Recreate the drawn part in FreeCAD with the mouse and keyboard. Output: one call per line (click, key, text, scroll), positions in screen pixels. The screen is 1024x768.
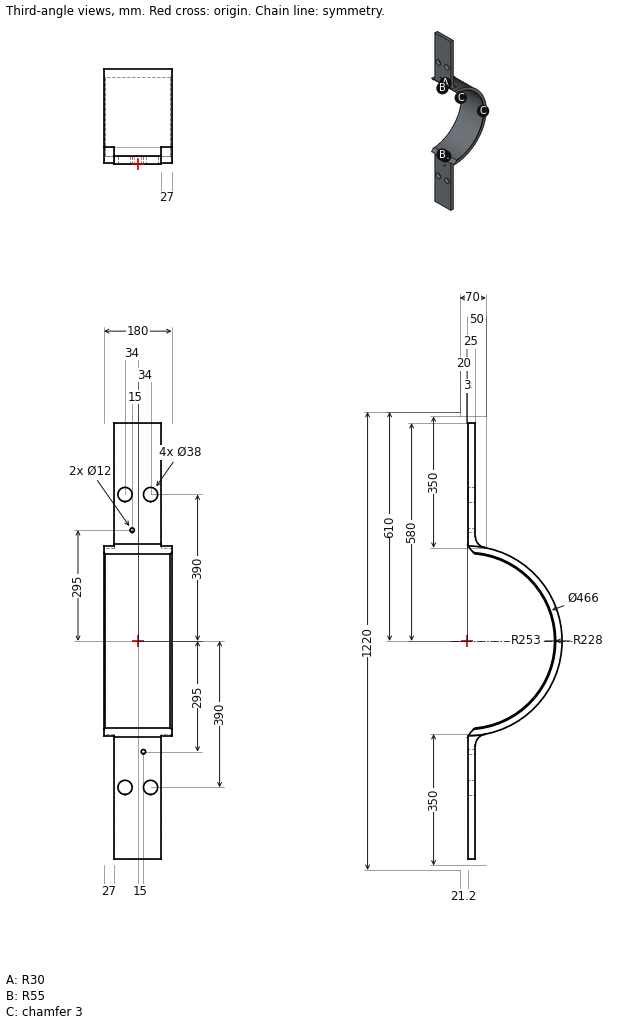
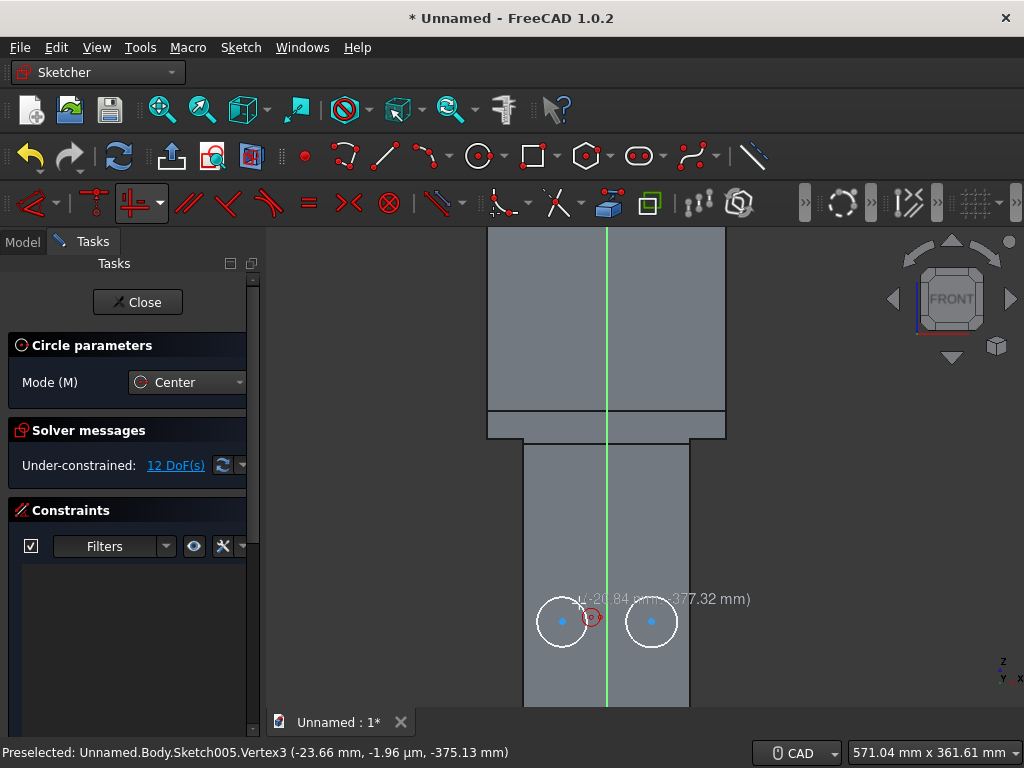
scroll(563, 624, down, 6)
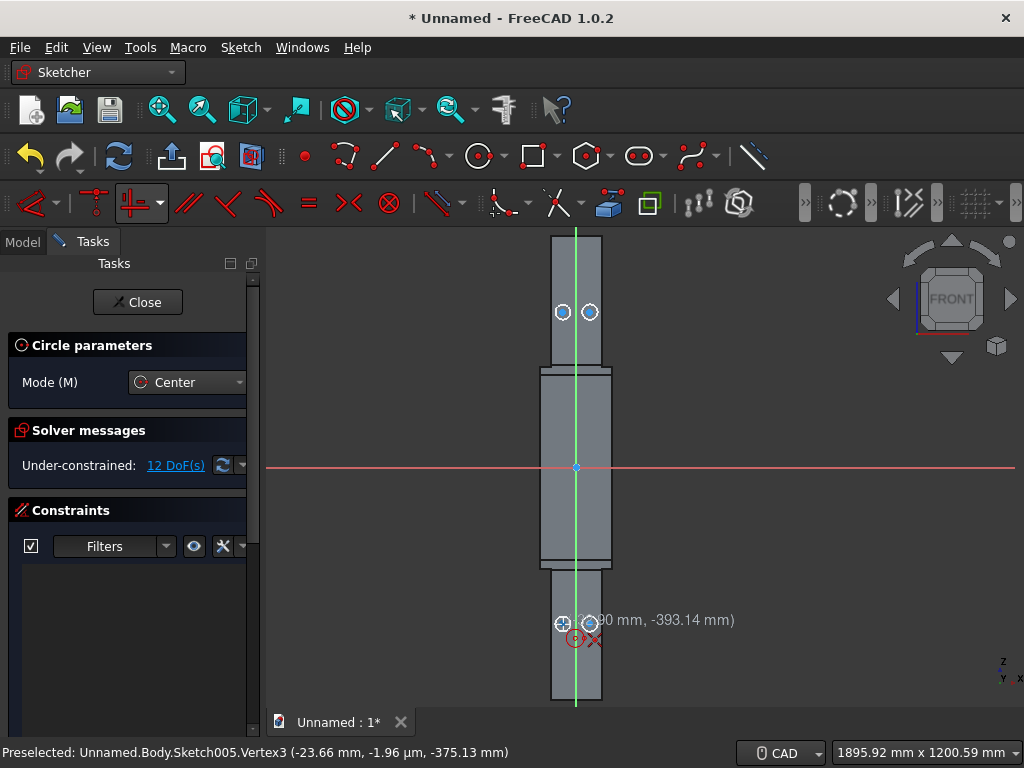
scroll(570, 350, up, 12)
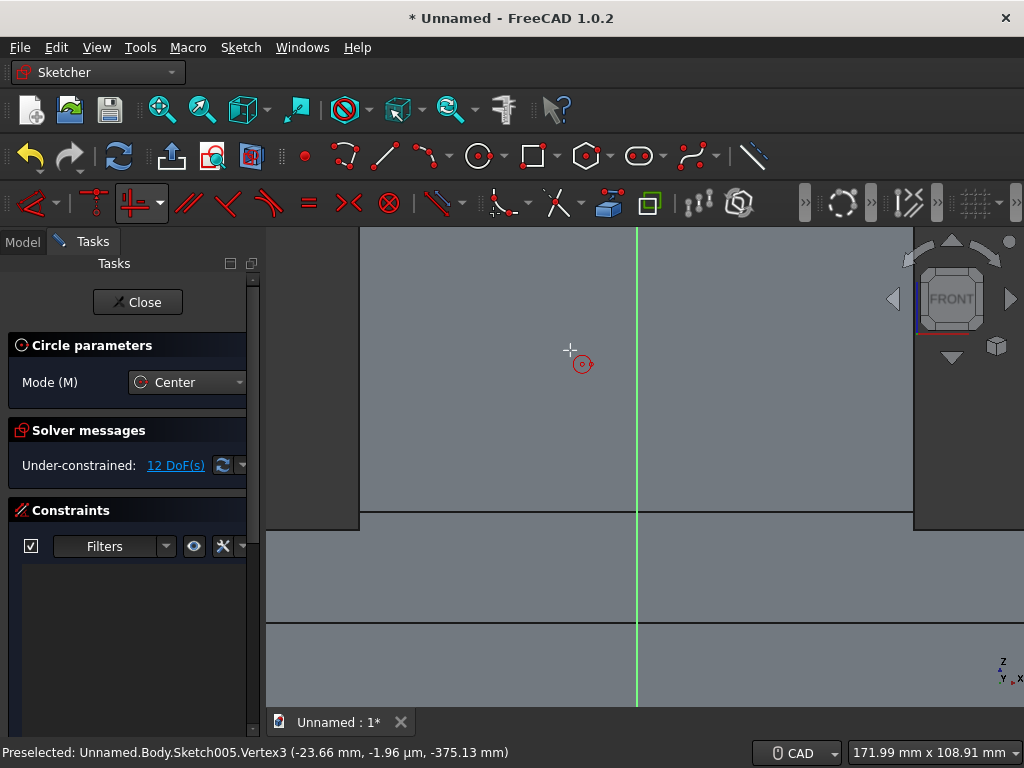
scroll(570, 349, down, 12)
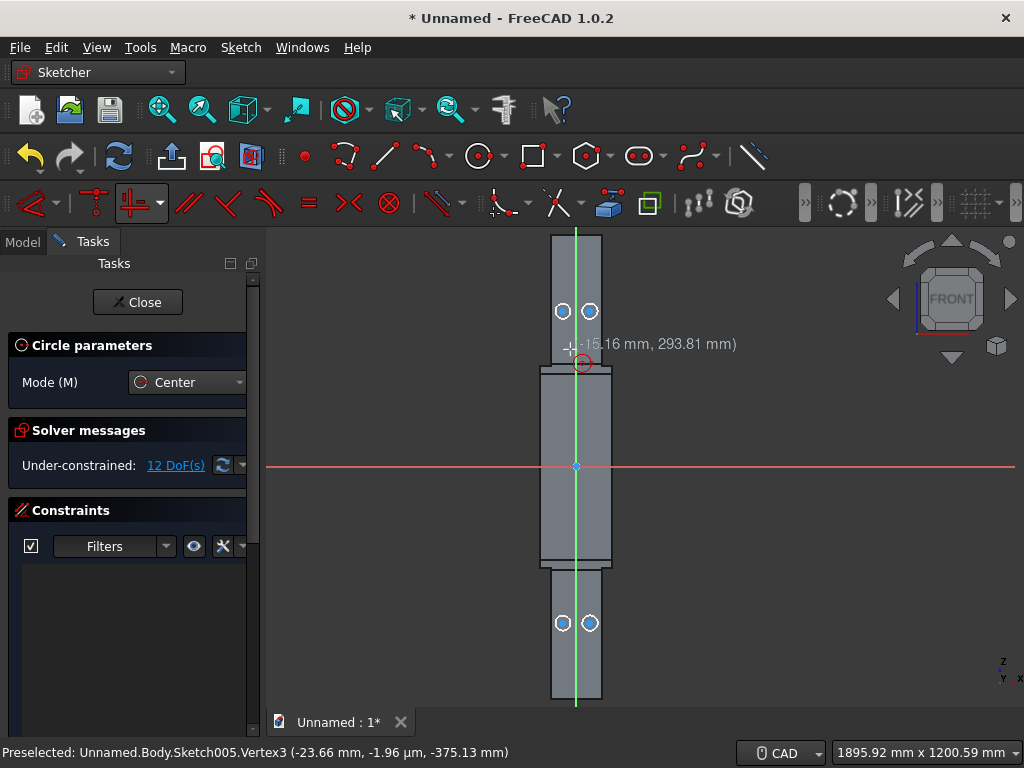
scroll(570, 349, up, 5)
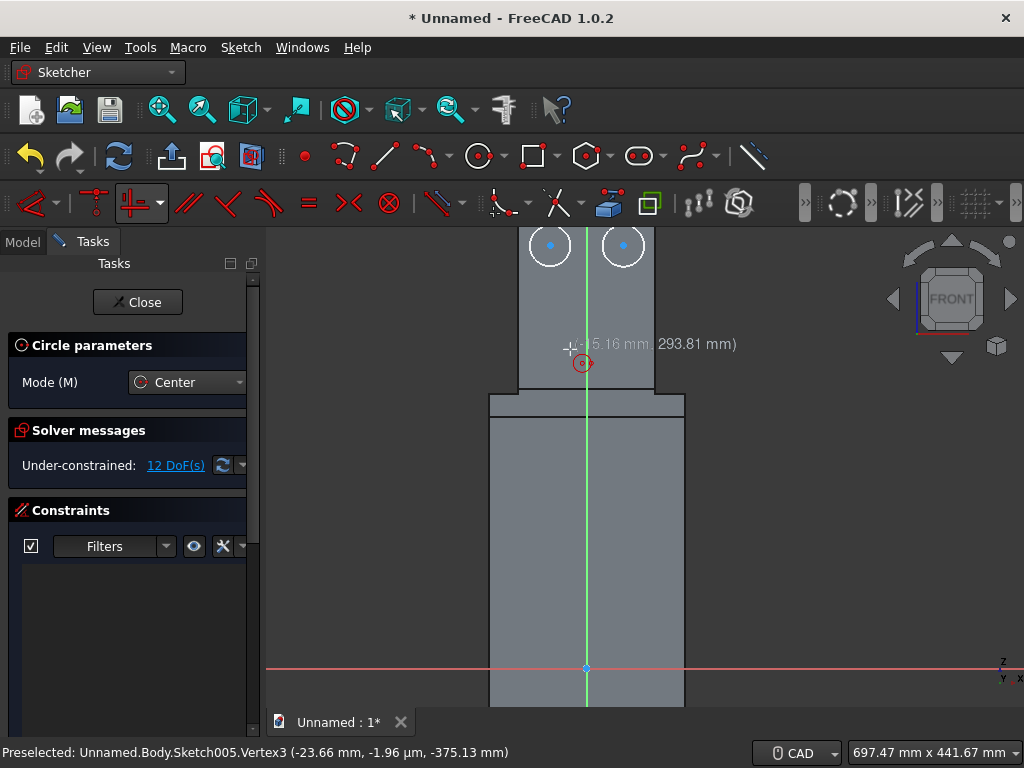
click(570, 348)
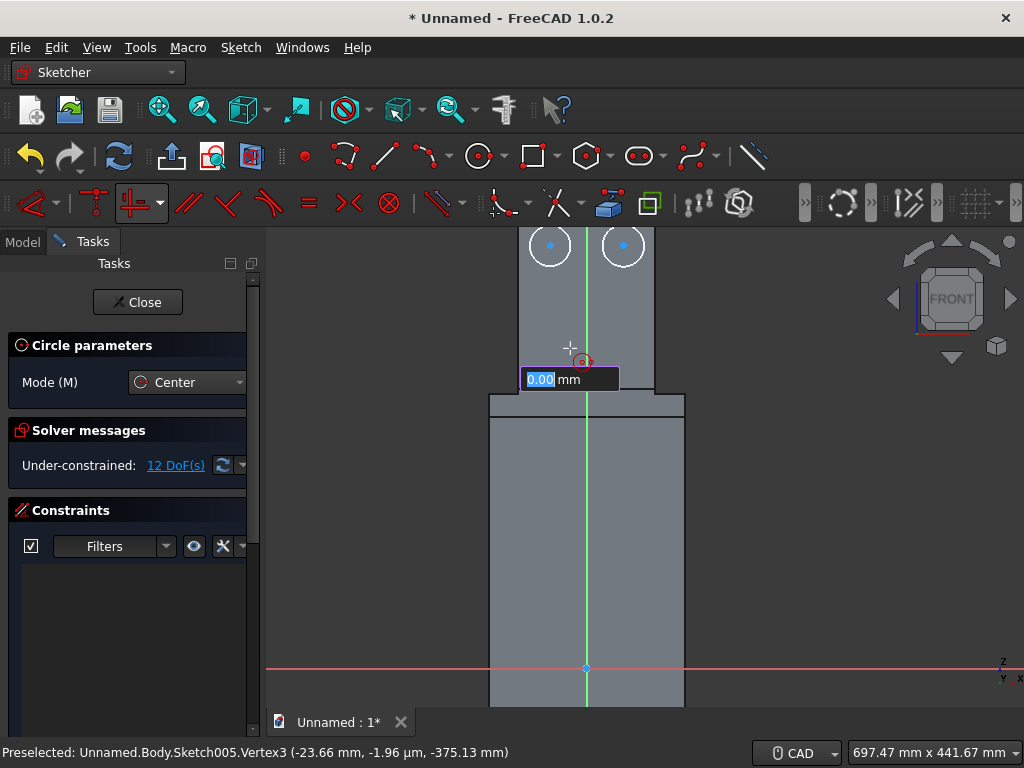
scroll(566, 344, up, 5)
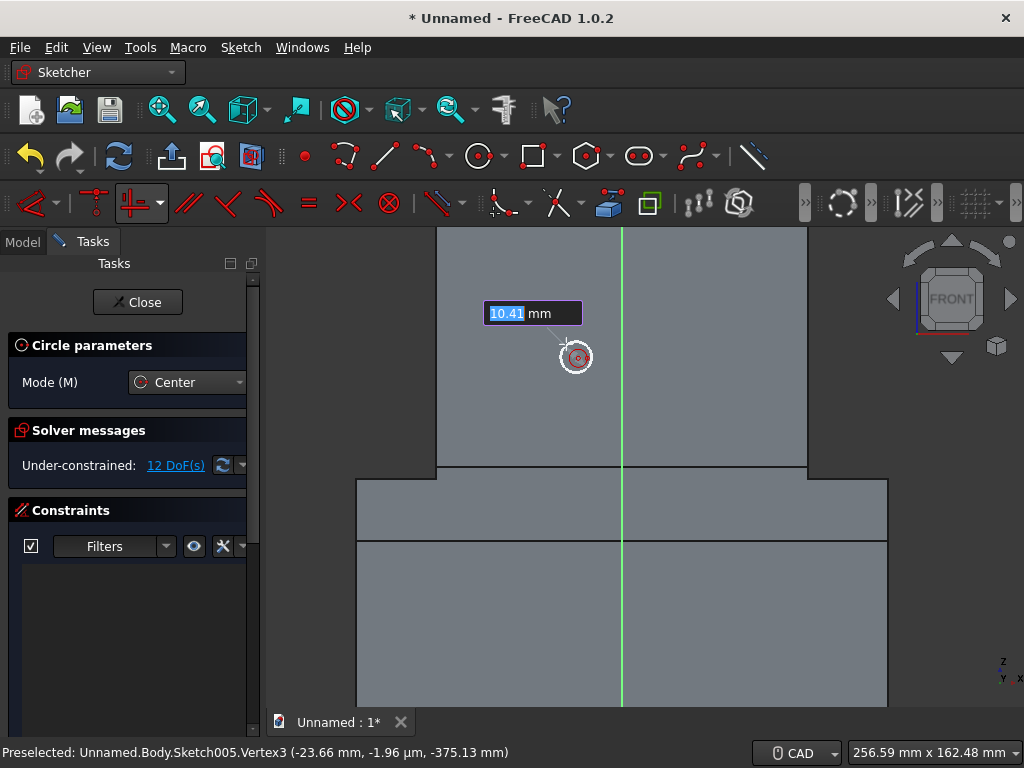
click(565, 342)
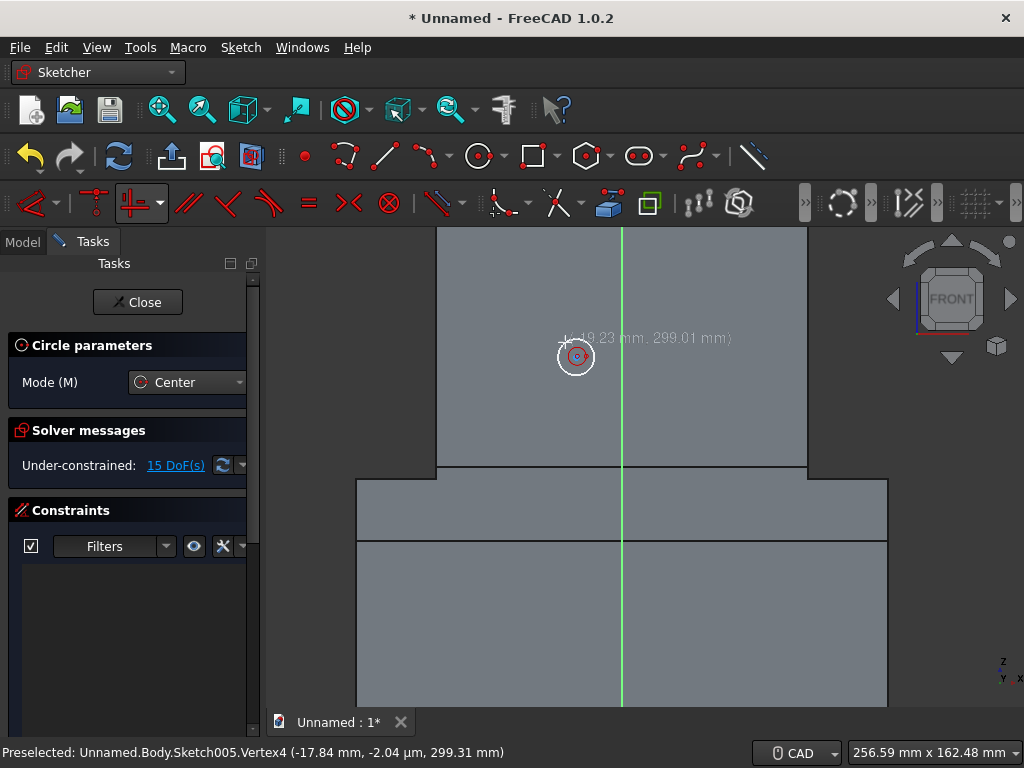
scroll(569, 348, down, 10)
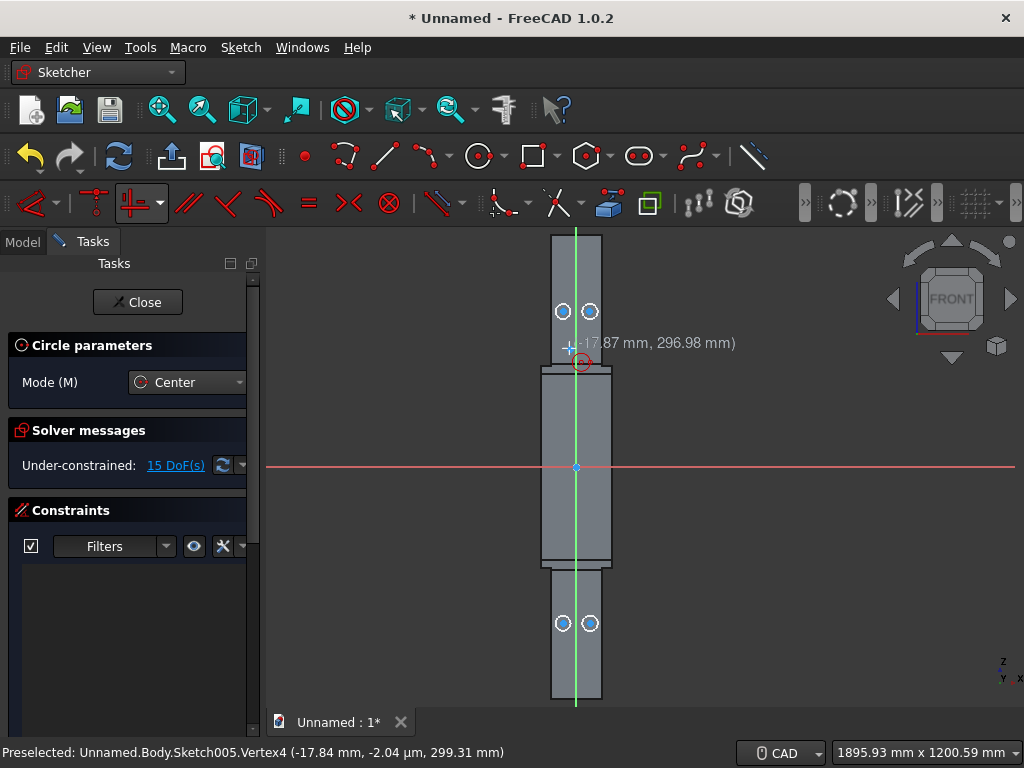
scroll(582, 585, up, 12)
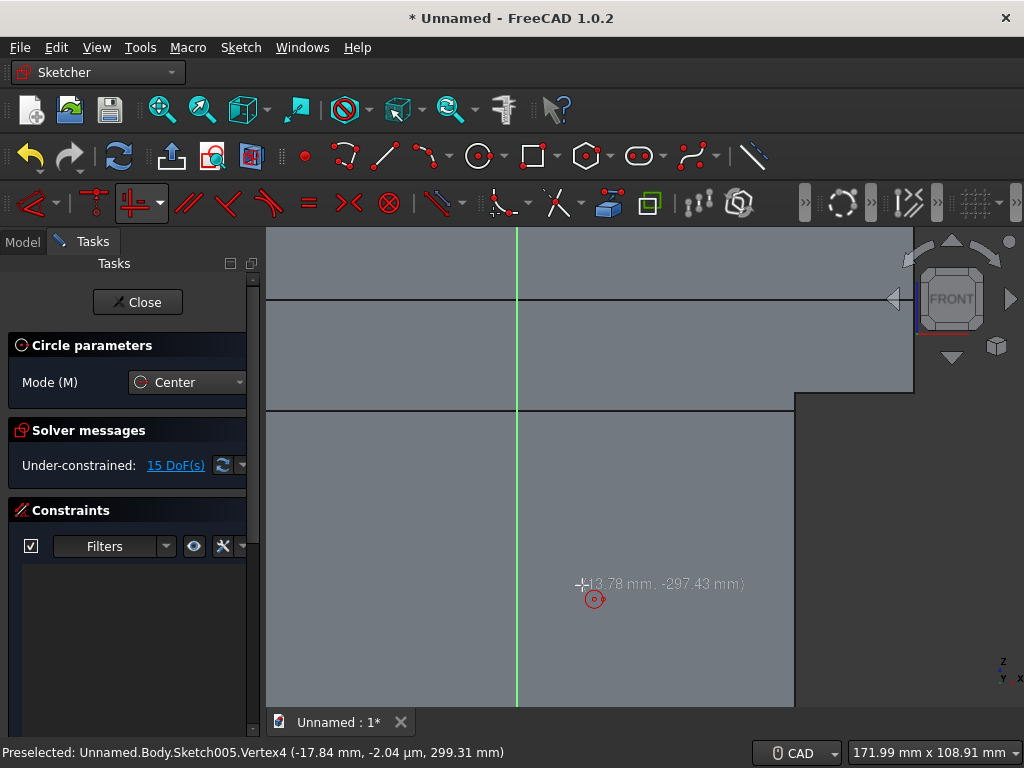
scroll(582, 586, down, 12)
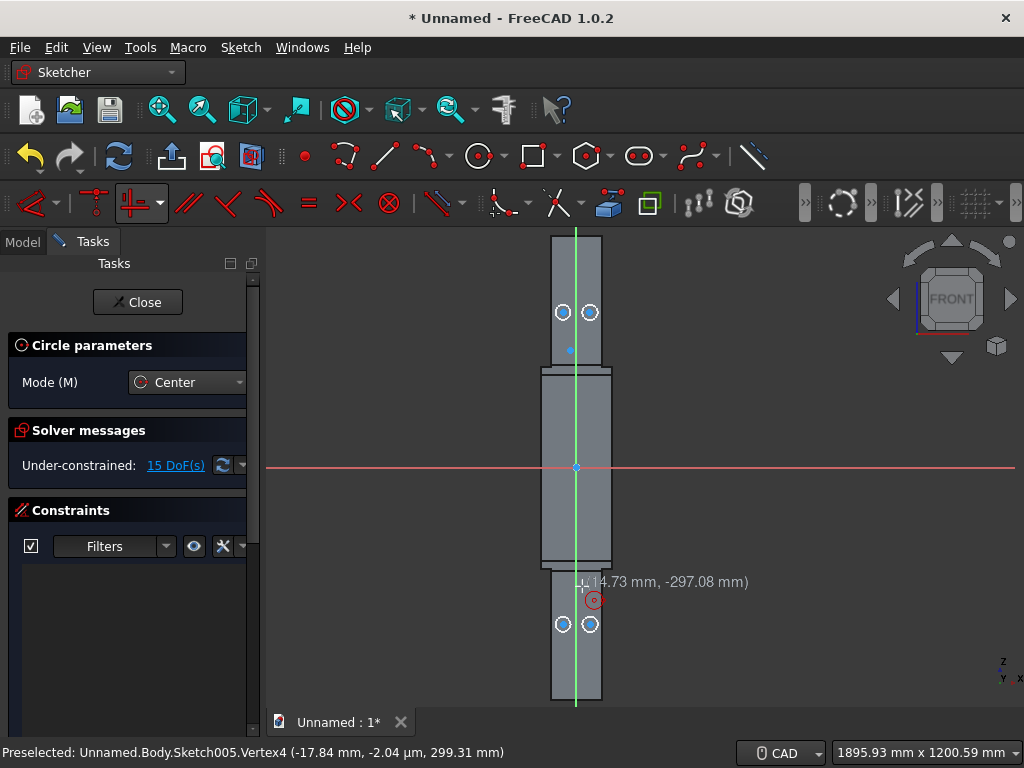
scroll(582, 586, up, 5)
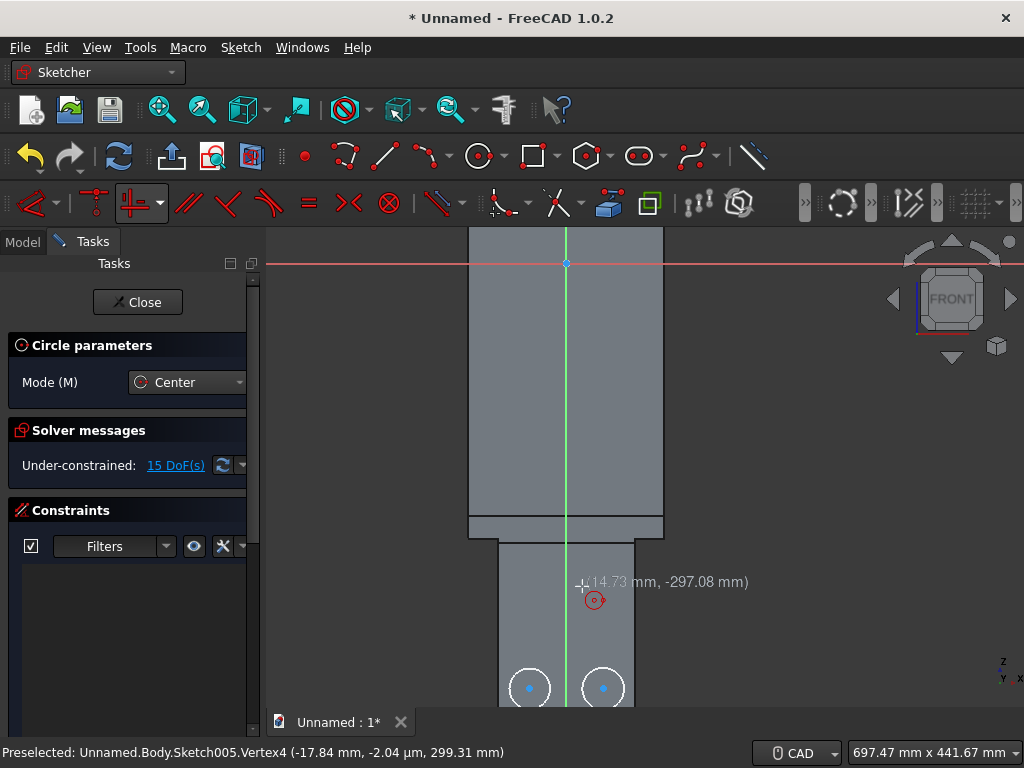
click(583, 585)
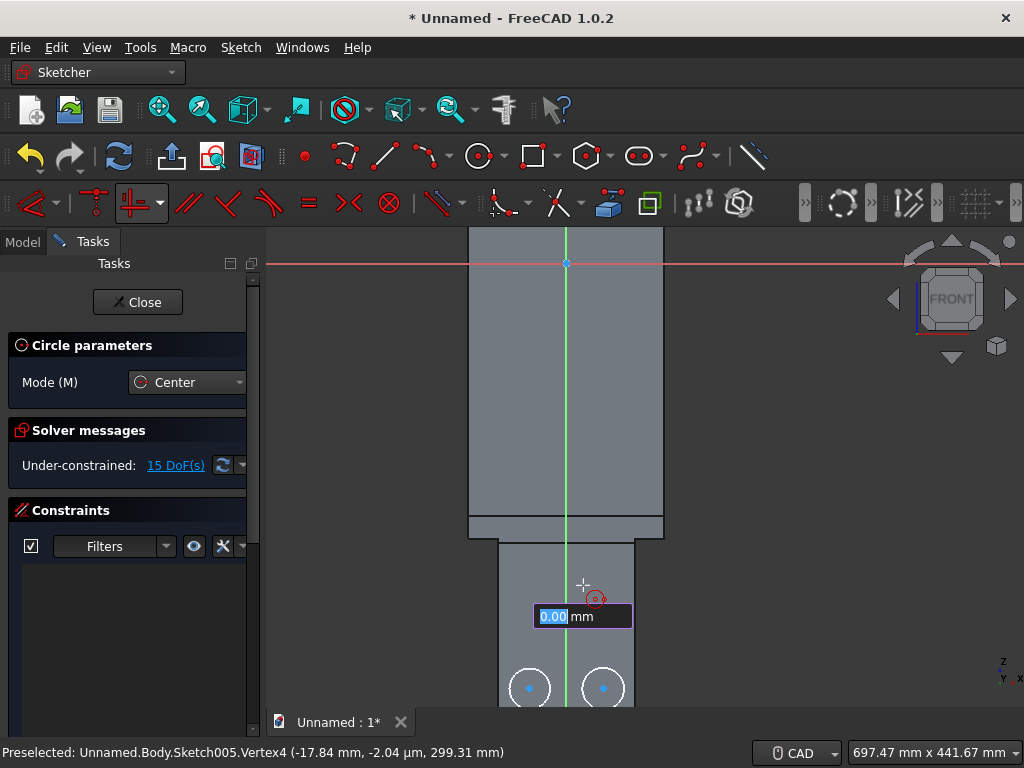
scroll(587, 580, up, 5)